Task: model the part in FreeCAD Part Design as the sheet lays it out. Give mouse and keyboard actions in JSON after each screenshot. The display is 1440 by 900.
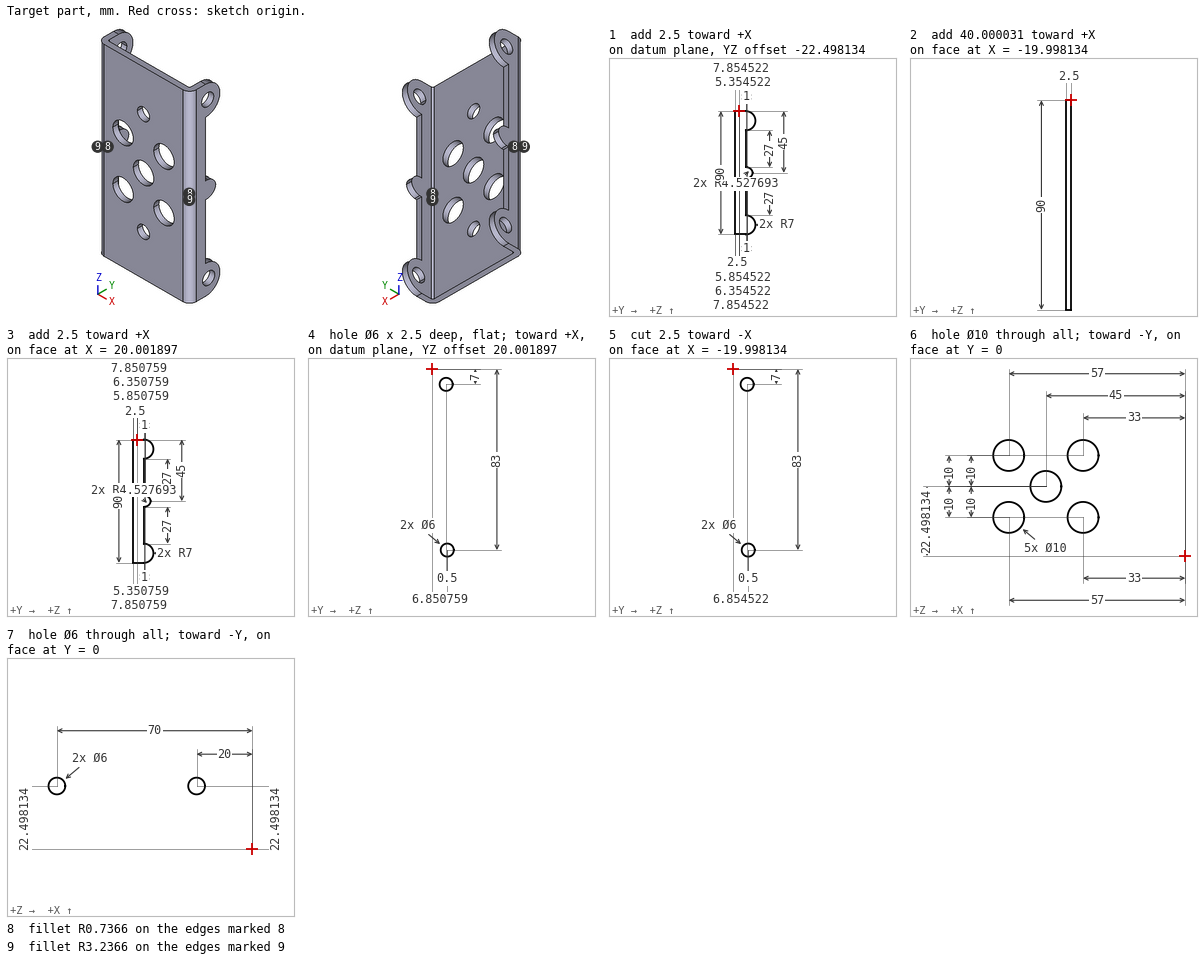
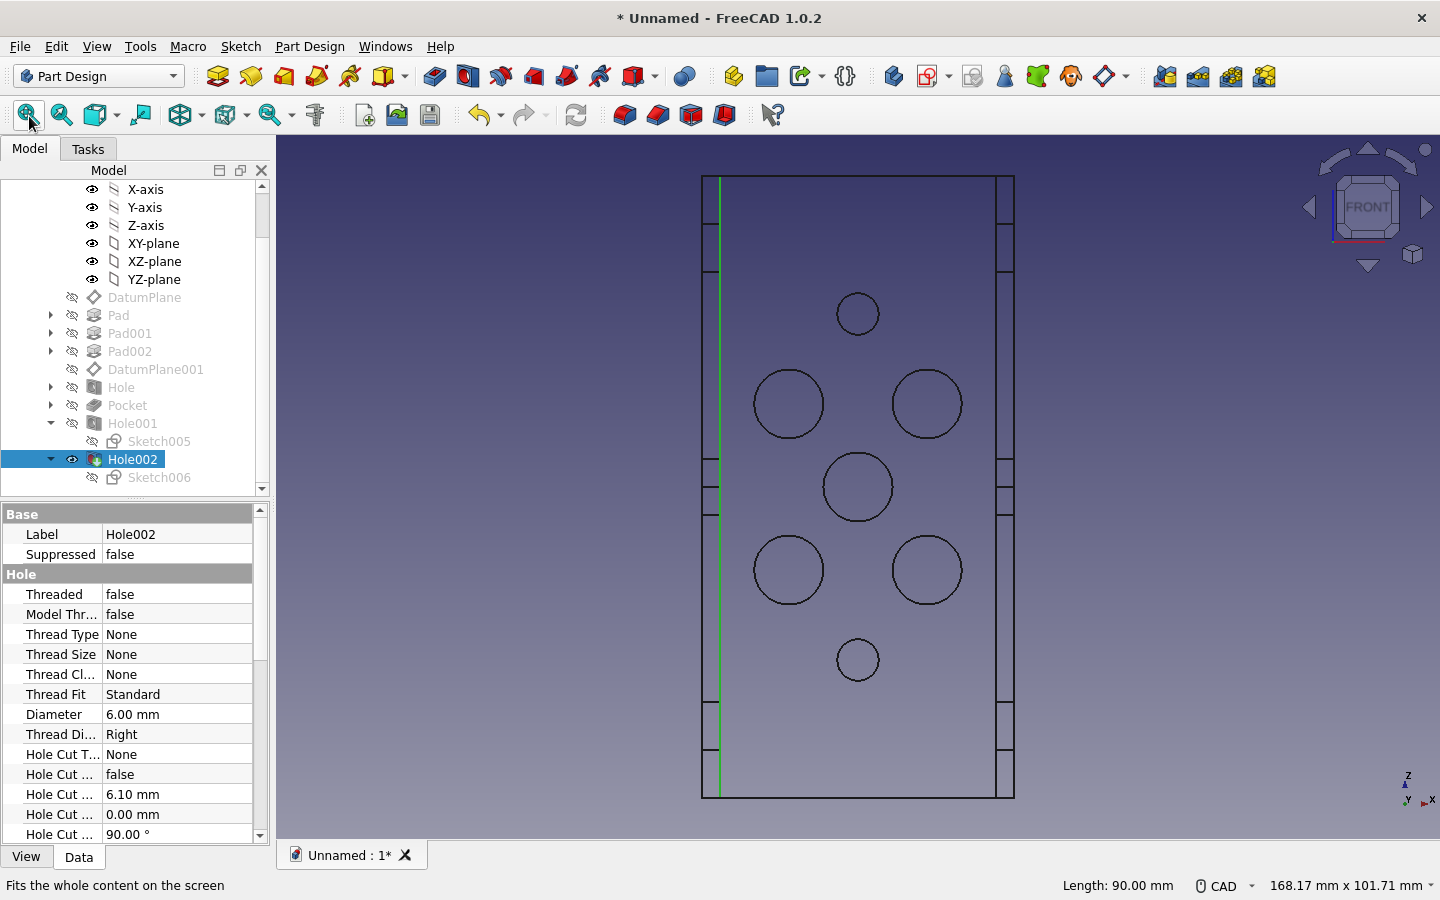
{"action": "left_click", "coordinate": [996, 486], "text": "ctrl"}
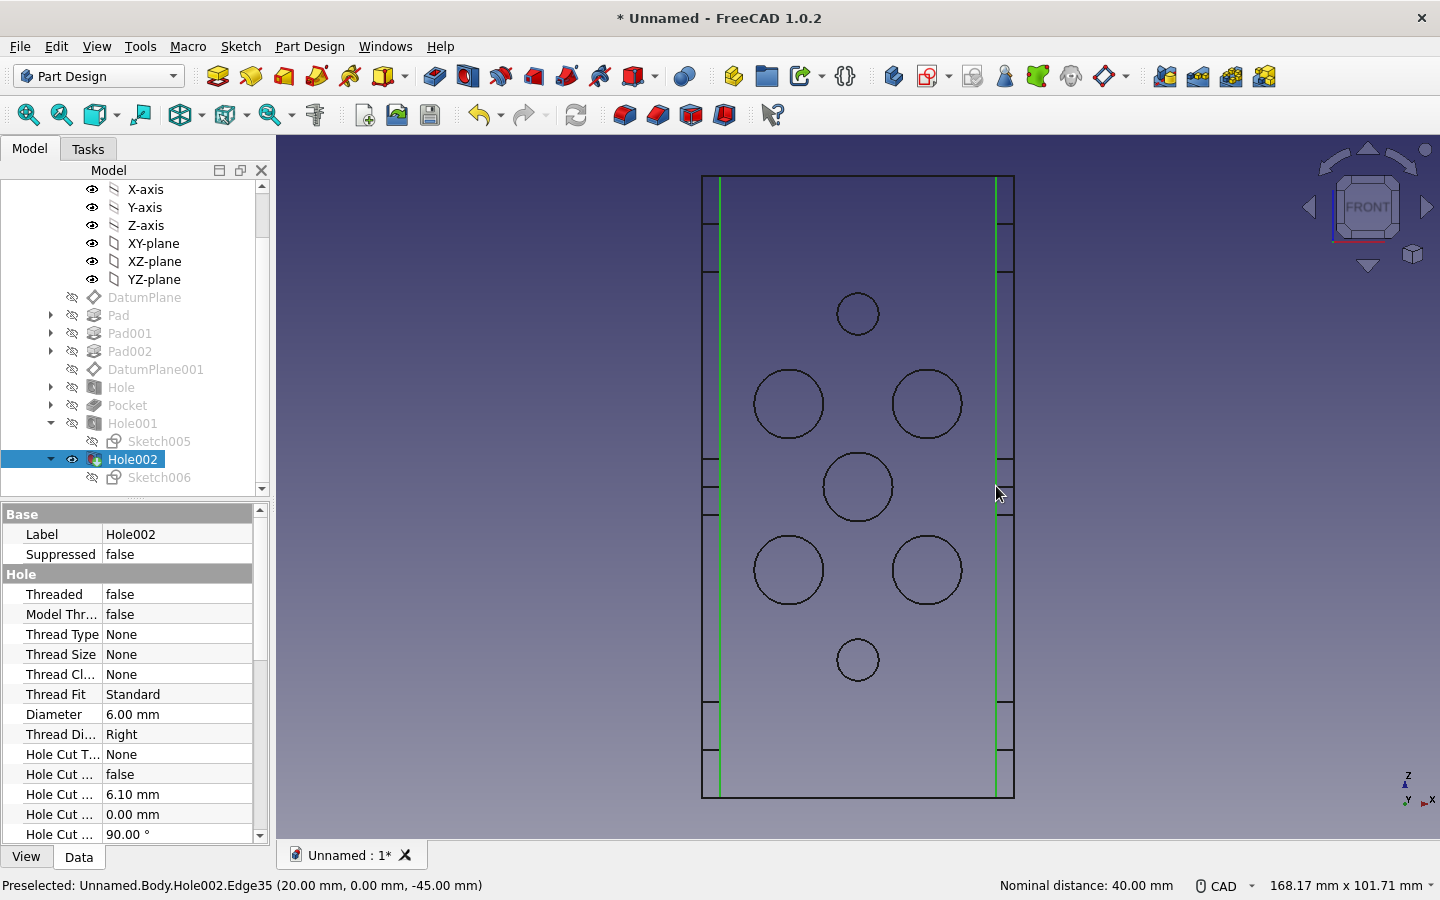
{"action": "key", "text": "v 1"}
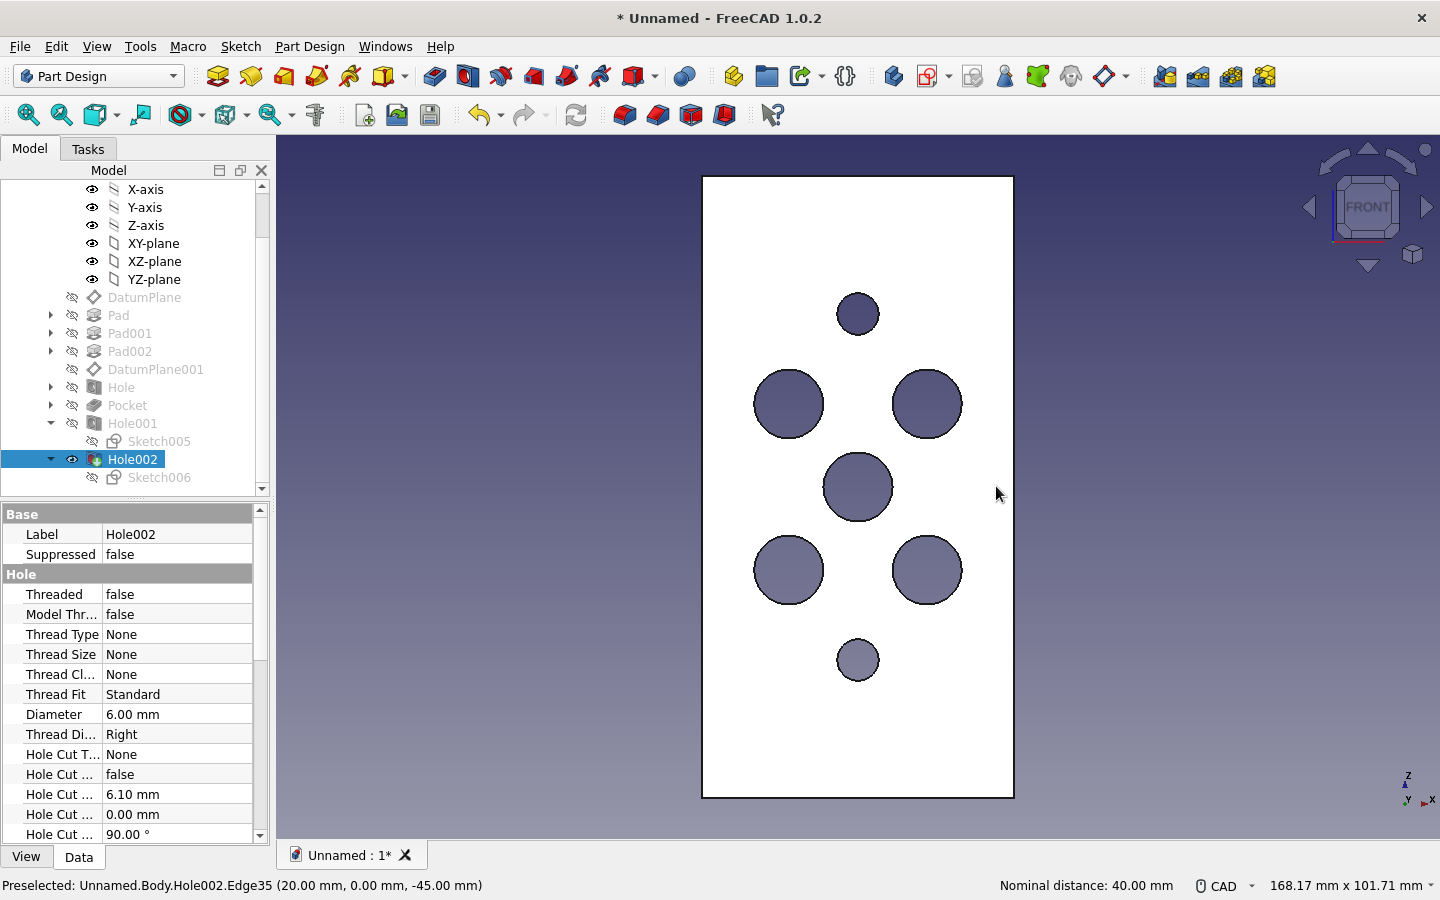
{"action": "left_click", "coordinate": [625, 116]}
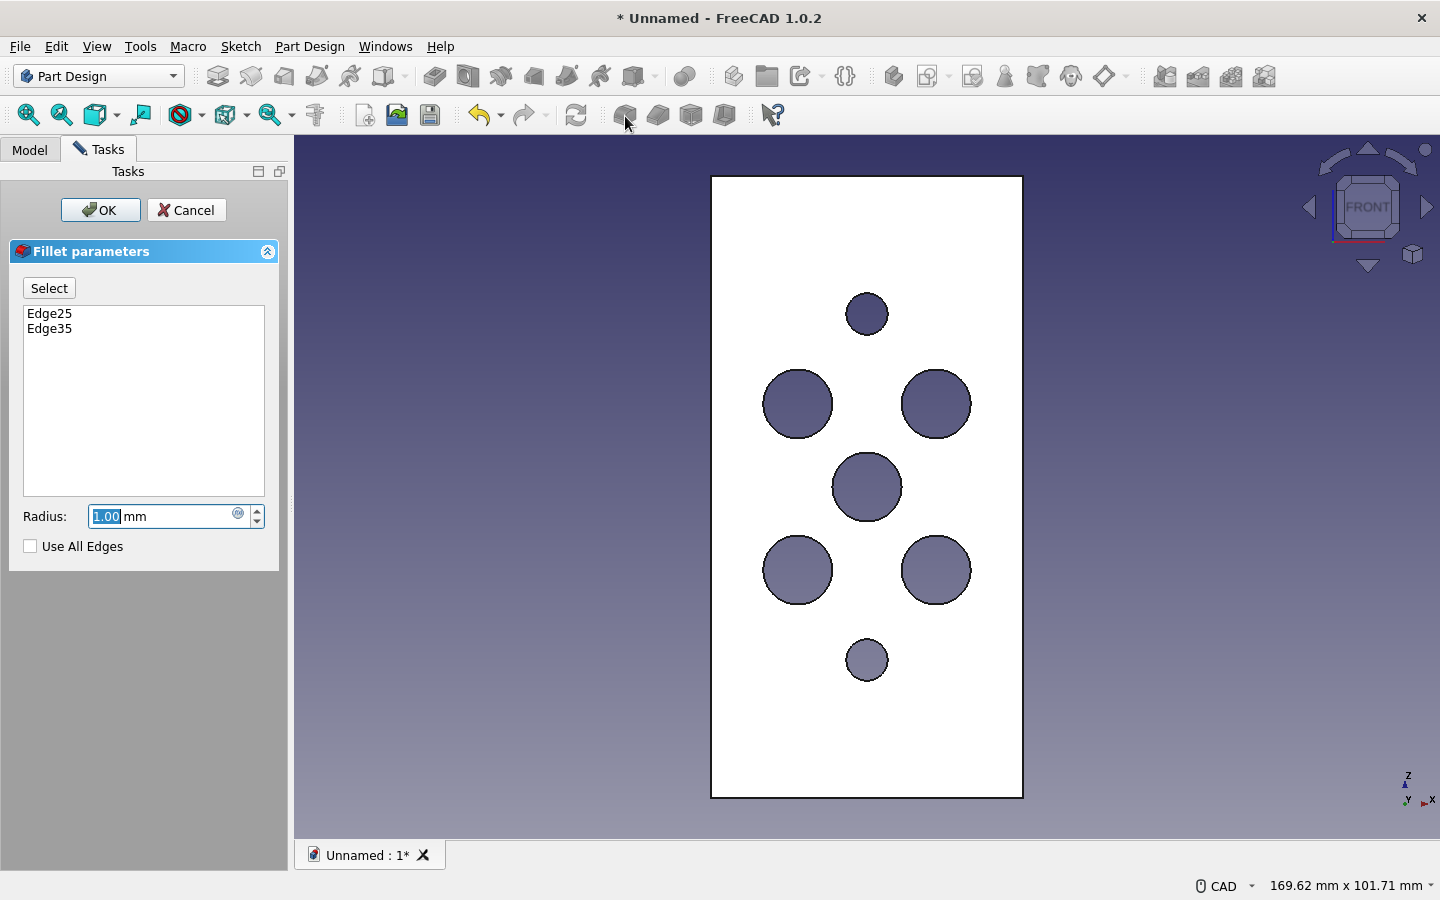
{"action": "type", "text": "0.7366"}
{"action": "key", "text": "Tab"}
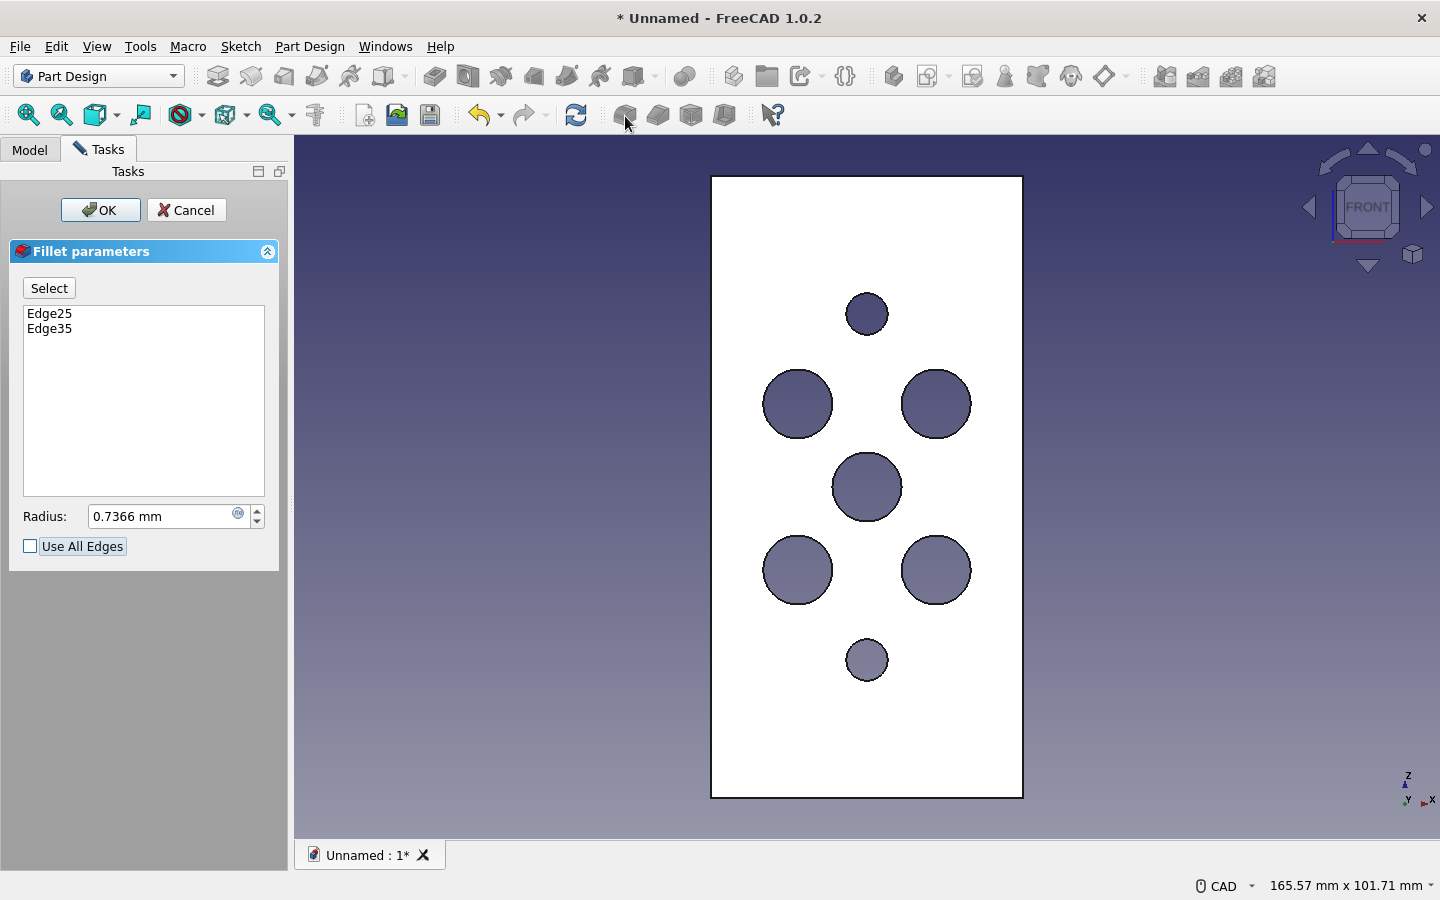
{"action": "left_click", "coordinate": [101, 210]}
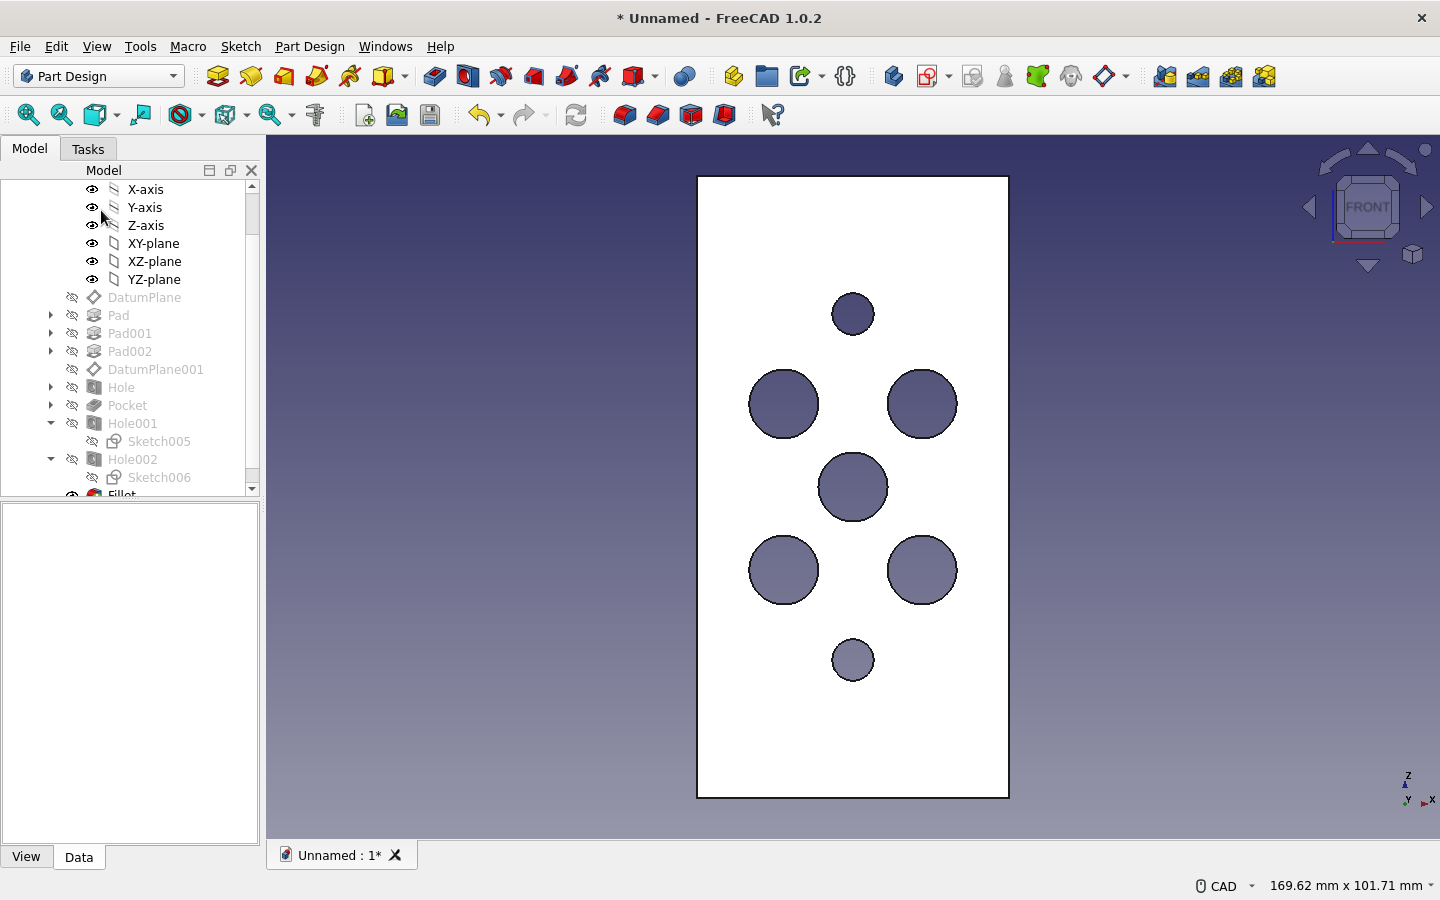
{"action": "left_click", "coordinate": [697, 486]}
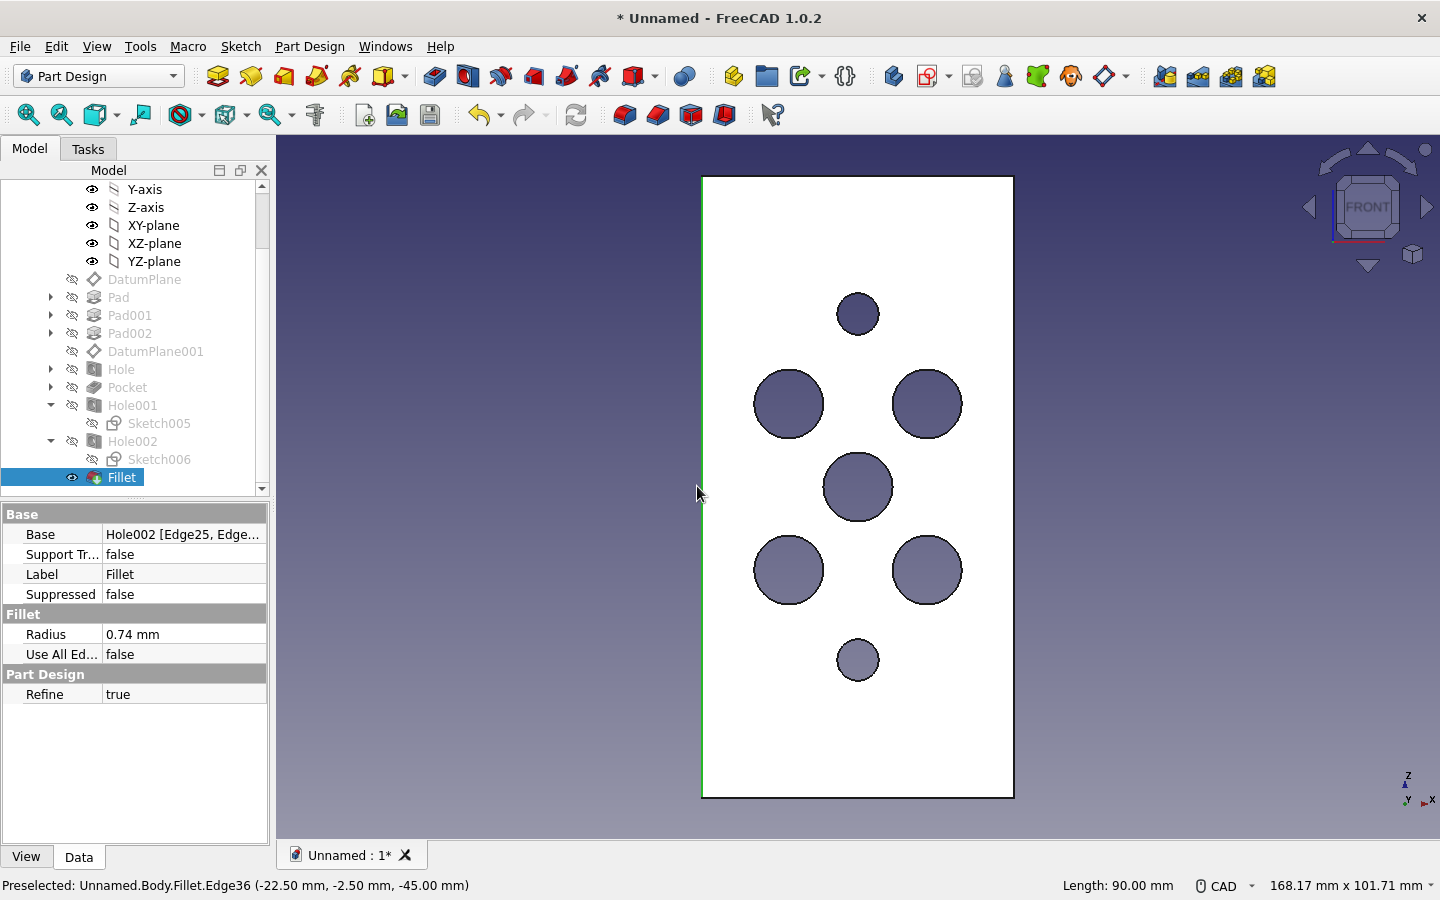
{"action": "left_click", "coordinate": [1014, 486], "text": "ctrl"}